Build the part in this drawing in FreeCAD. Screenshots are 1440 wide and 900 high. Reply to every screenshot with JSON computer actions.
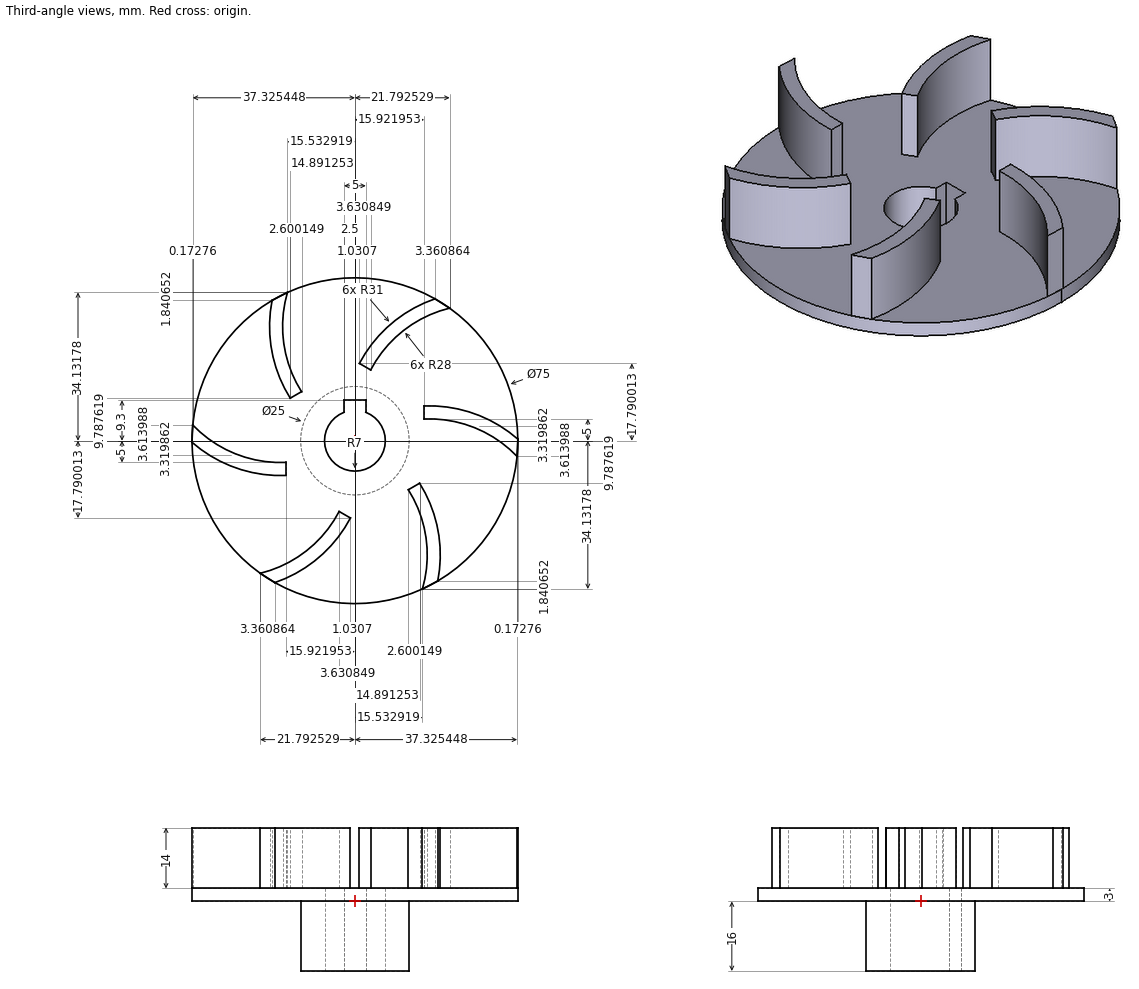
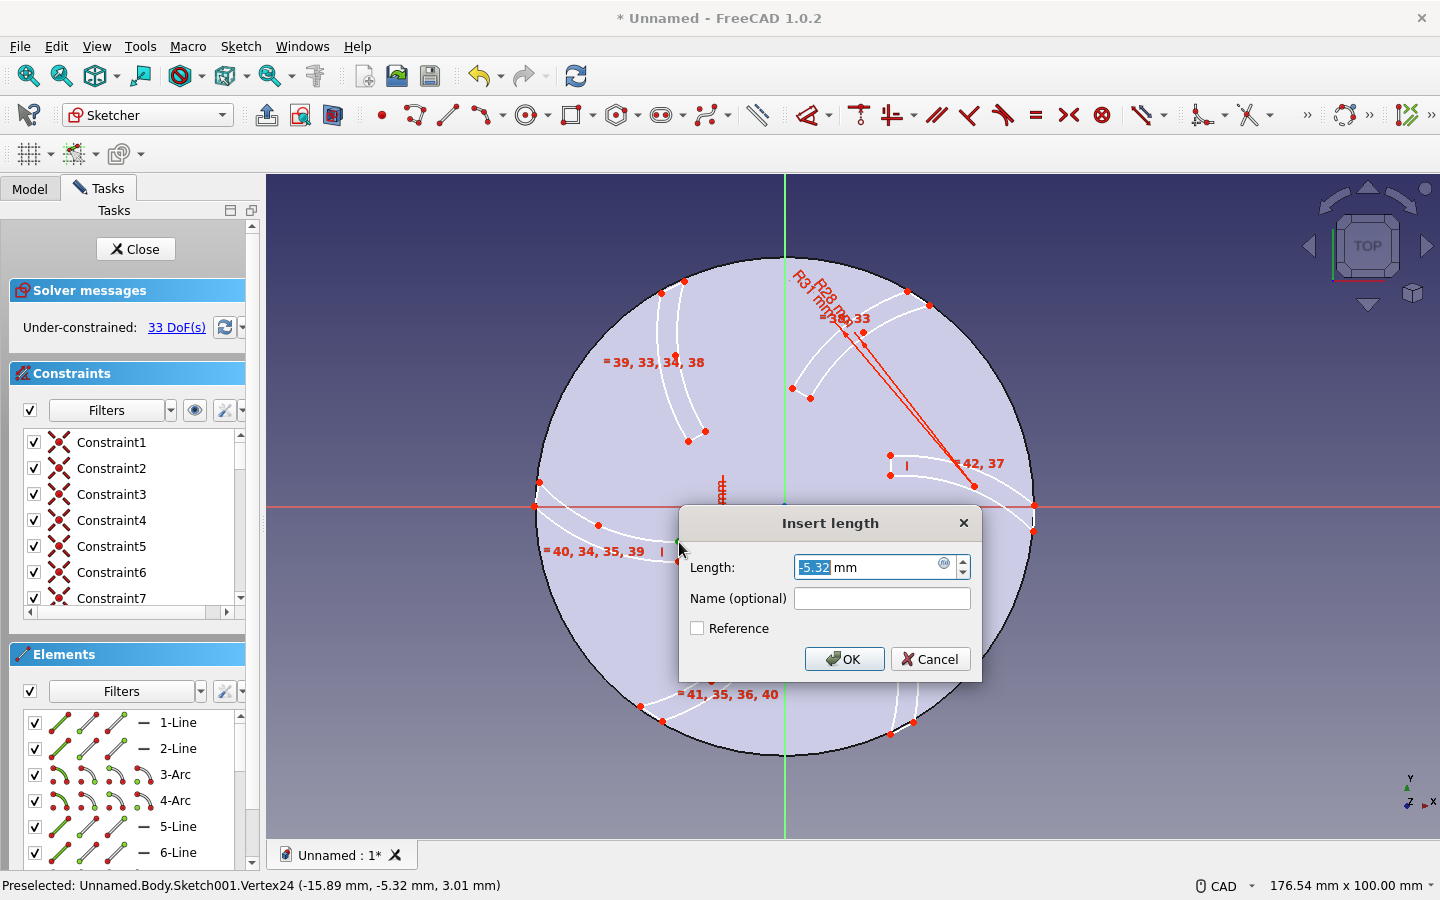
{"action": "type", "text": "-5"}
{"action": "key", "text": "Return"}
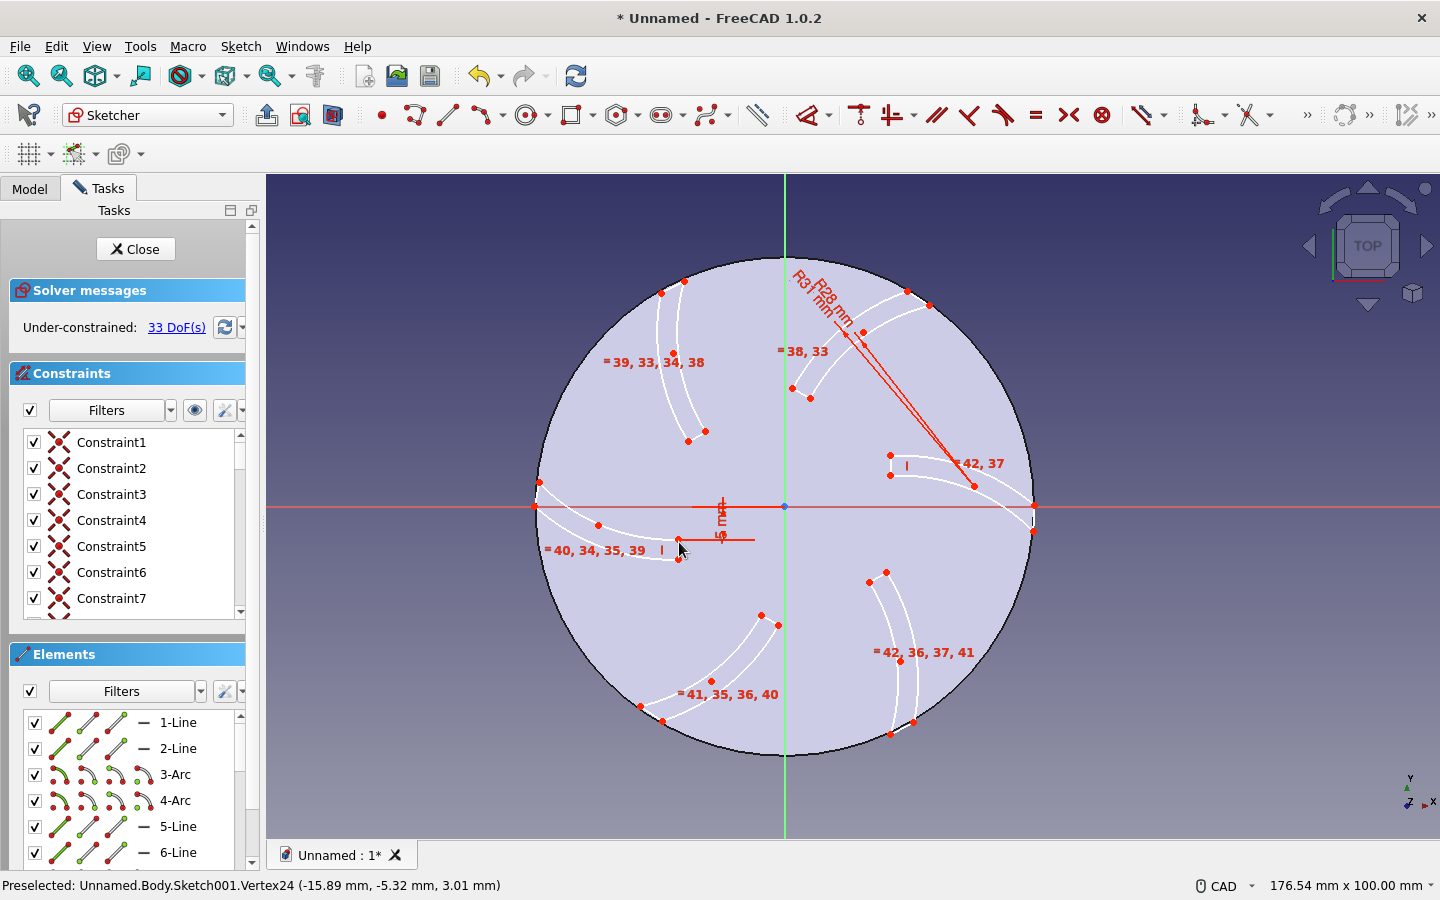
{"action": "left_click", "coordinate": [891, 476]}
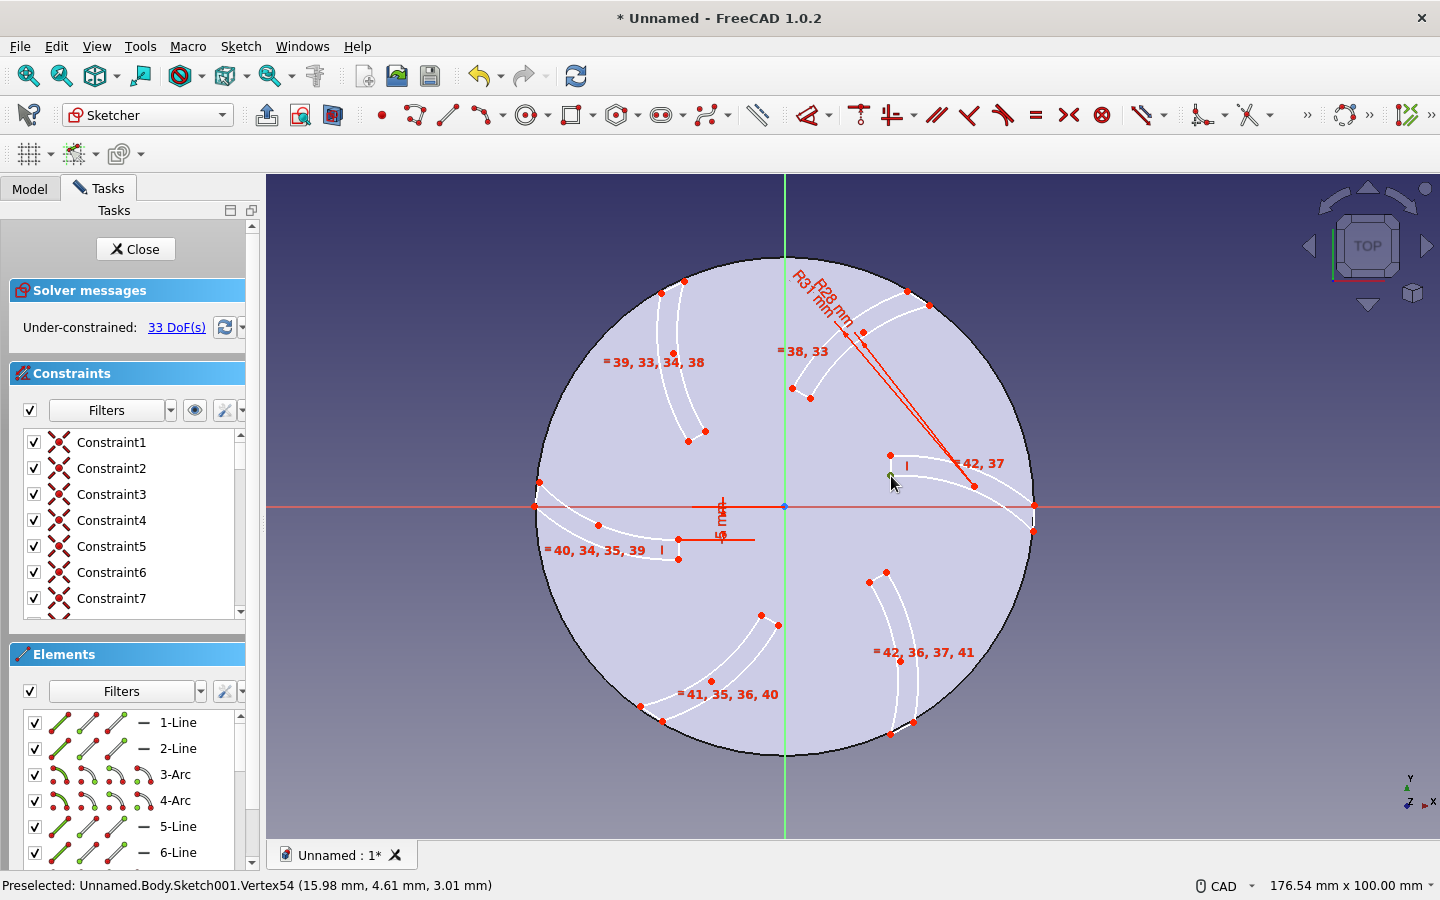
{"action": "key", "text": "i"}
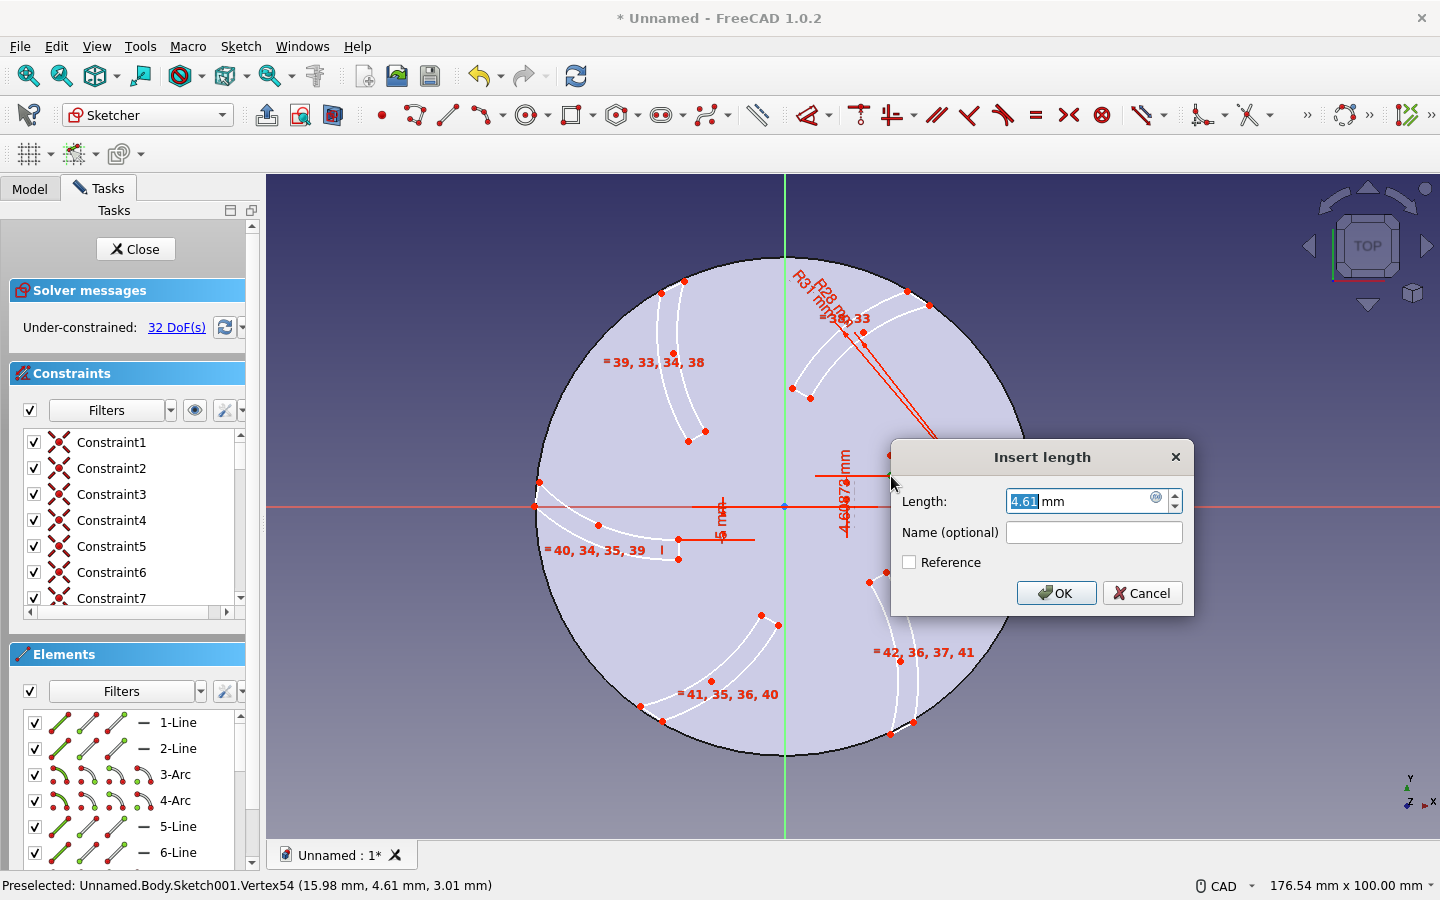
{"action": "type", "text": "5"}
{"action": "key", "text": "Return"}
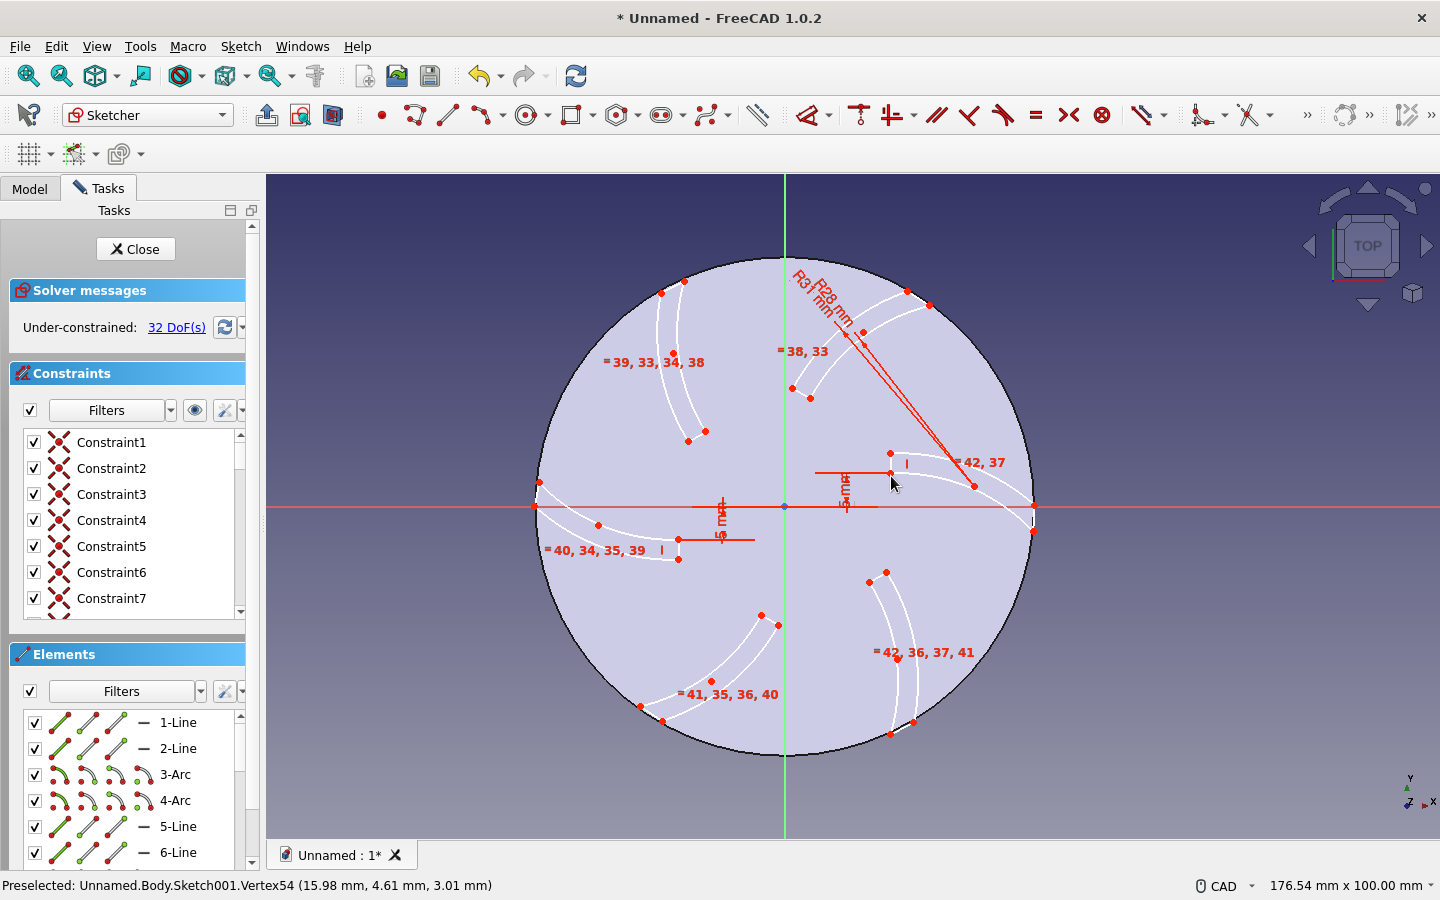
{"action": "scroll", "coordinate": [793, 389], "scroll_direction": "up", "scroll_amount": 9}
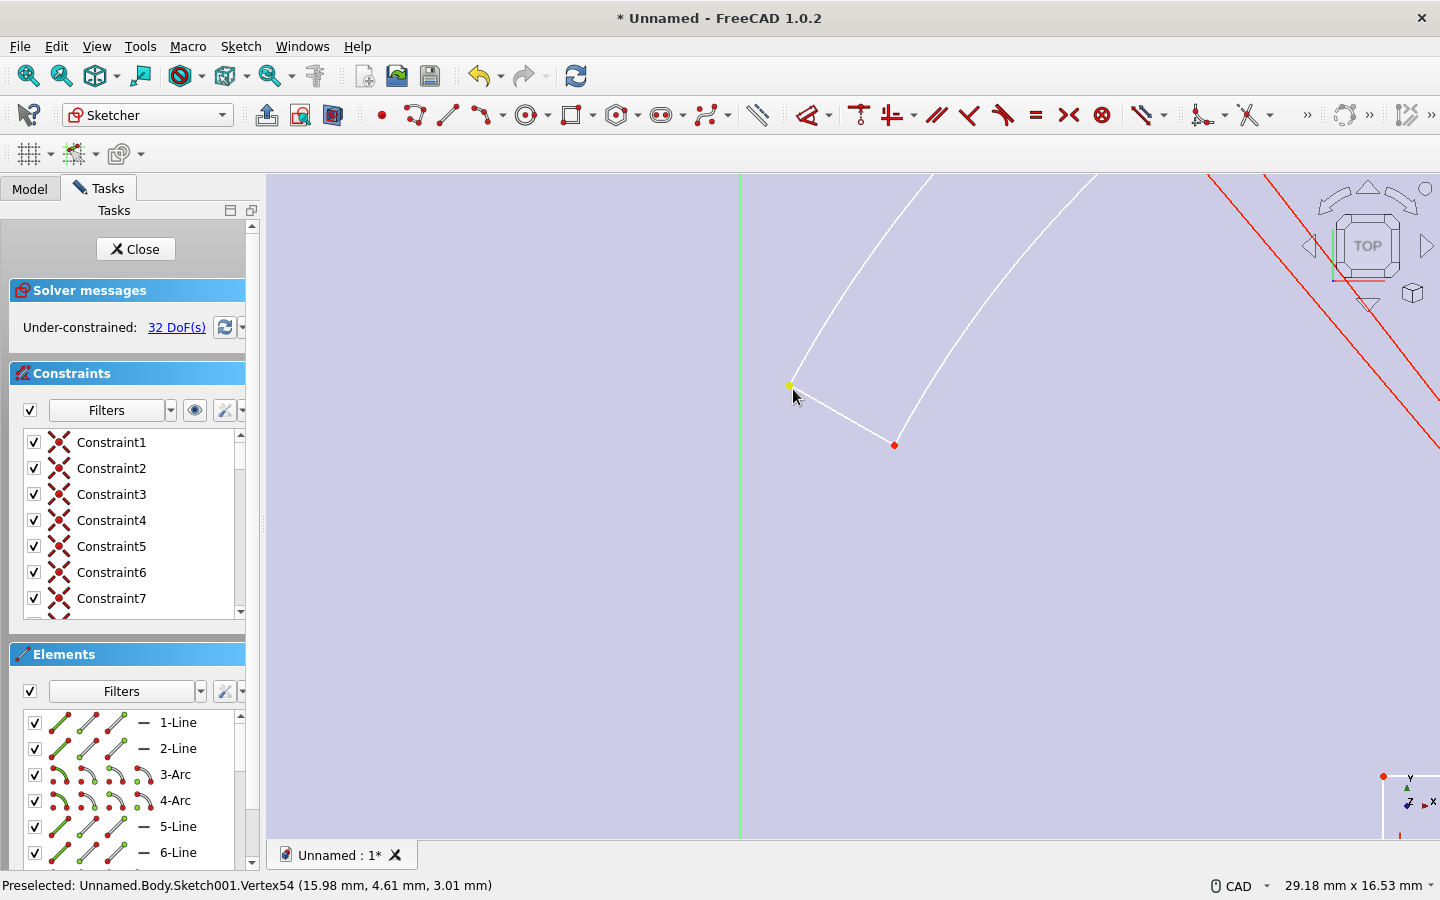
{"action": "left_click", "coordinate": [790, 385]}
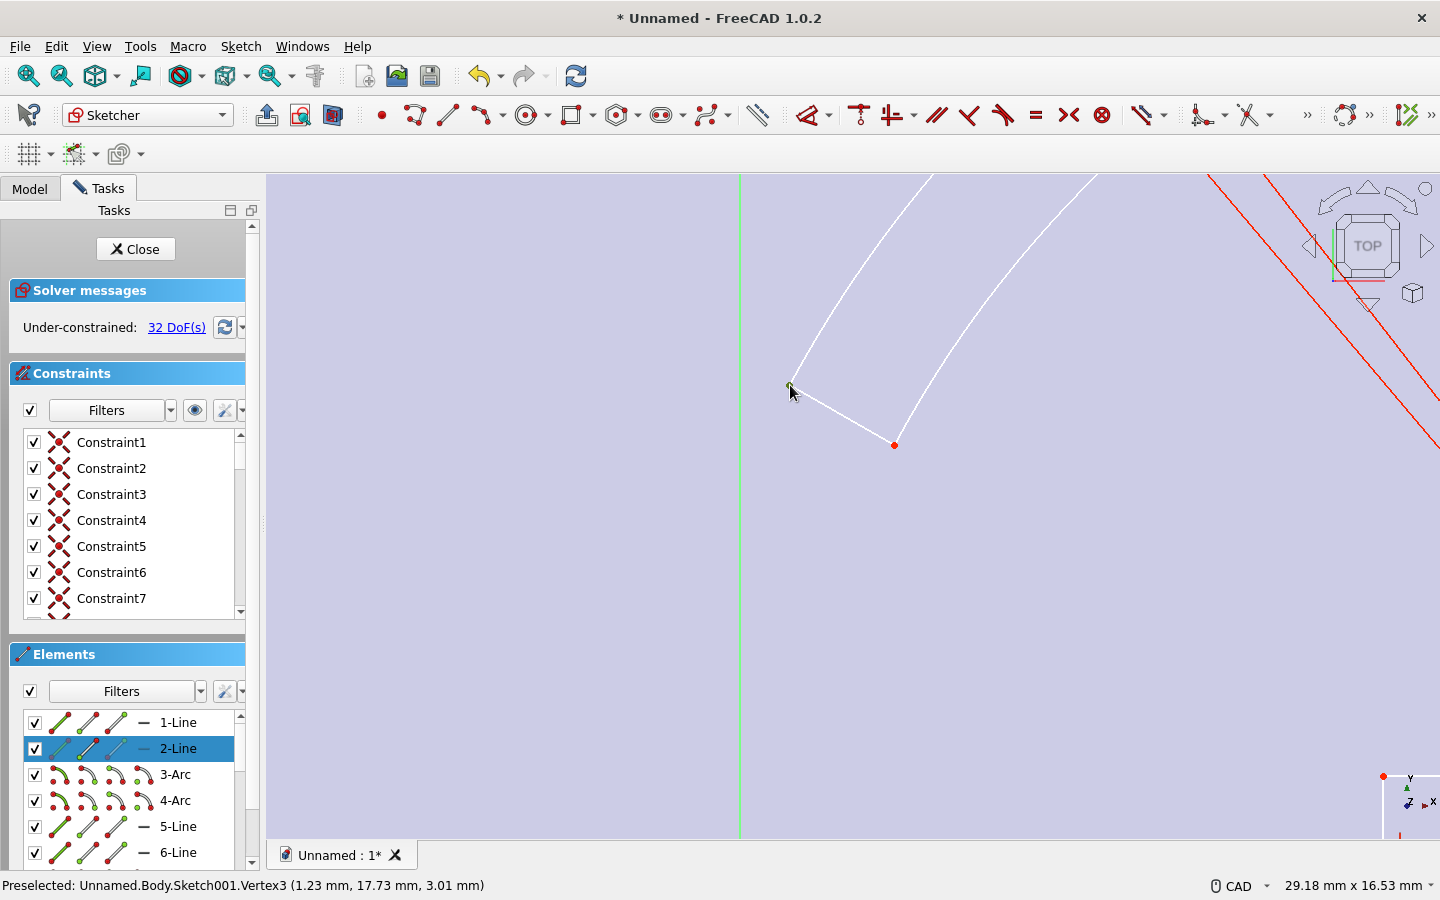
{"action": "key", "text": "l"}